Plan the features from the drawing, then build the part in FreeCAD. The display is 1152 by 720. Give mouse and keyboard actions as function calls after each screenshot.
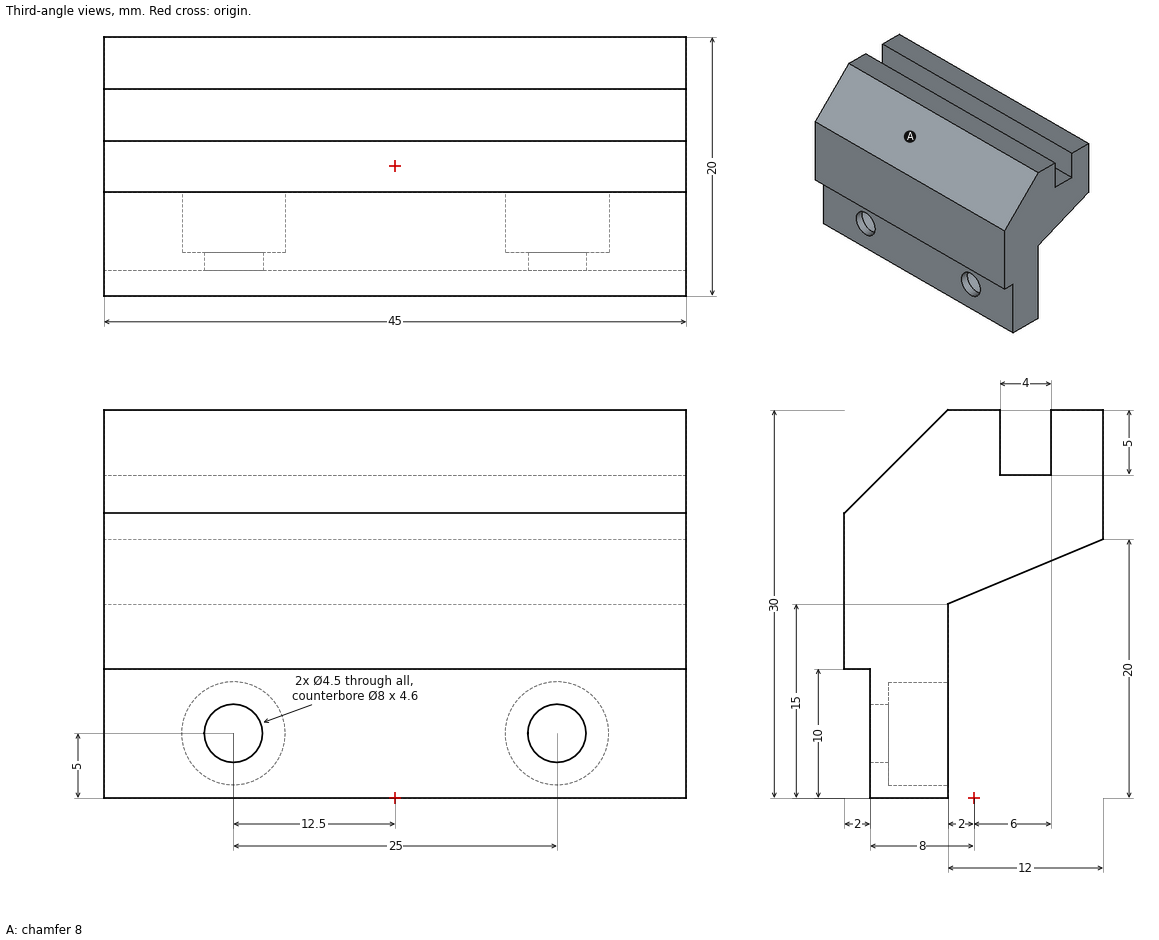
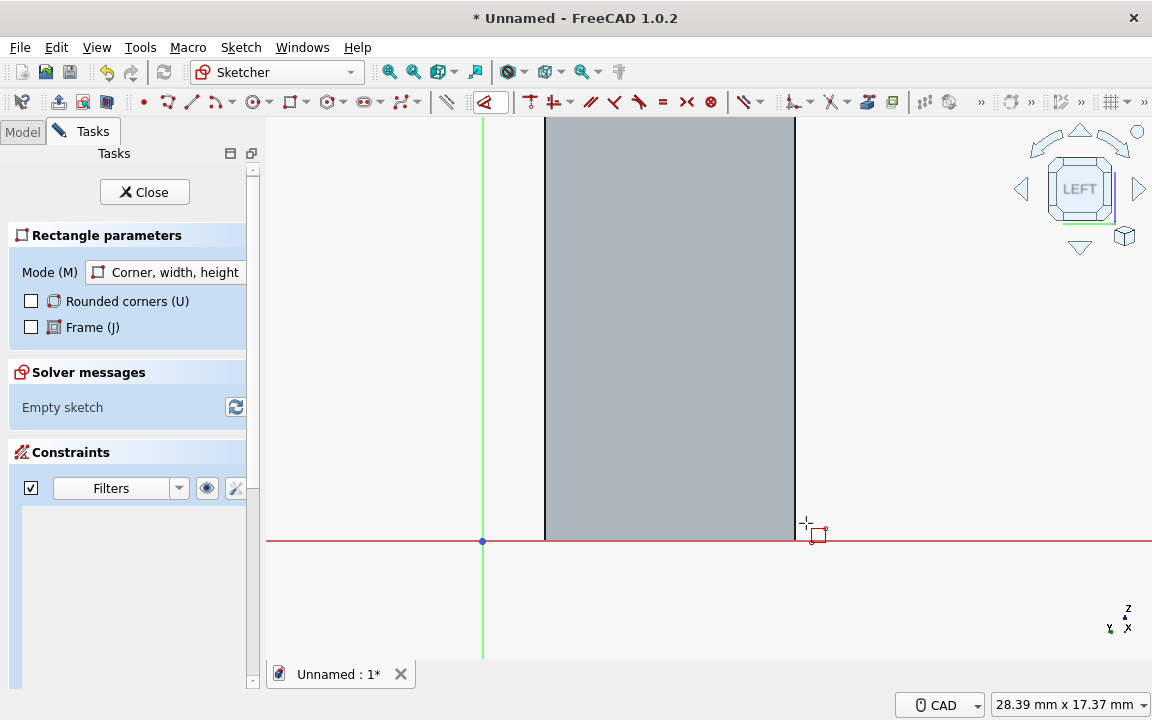
click(732, 229)
click(795, 541)
key(Escape)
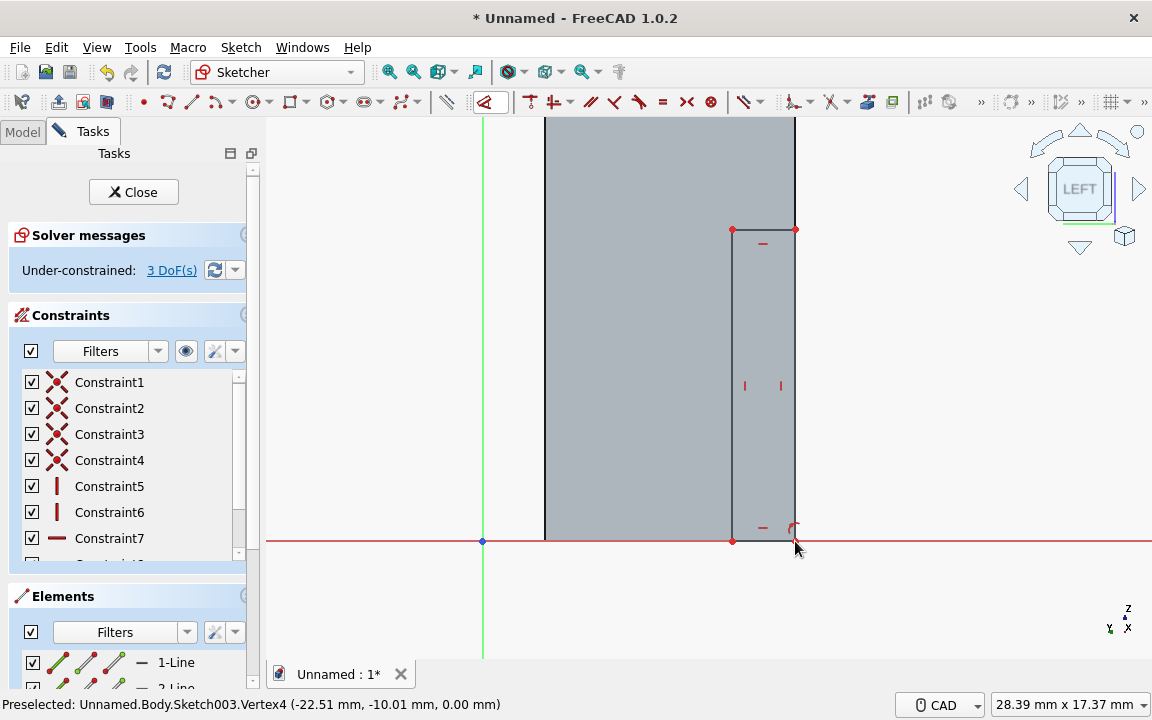
click(751, 541)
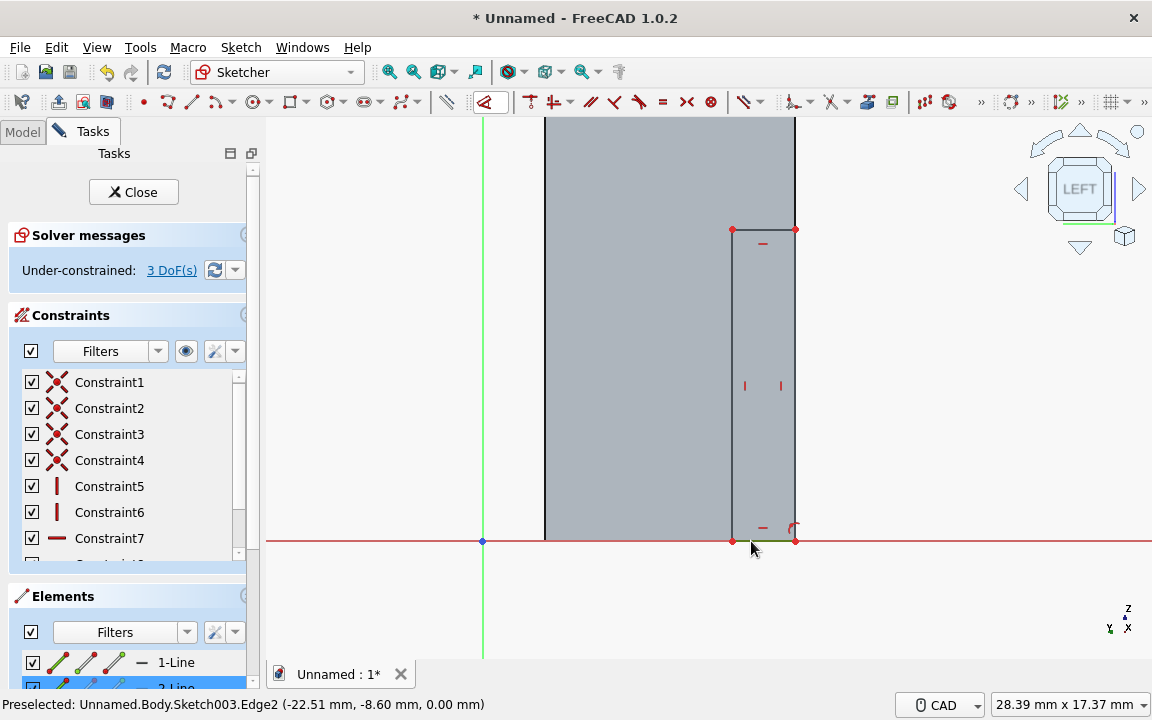
click(502, 102)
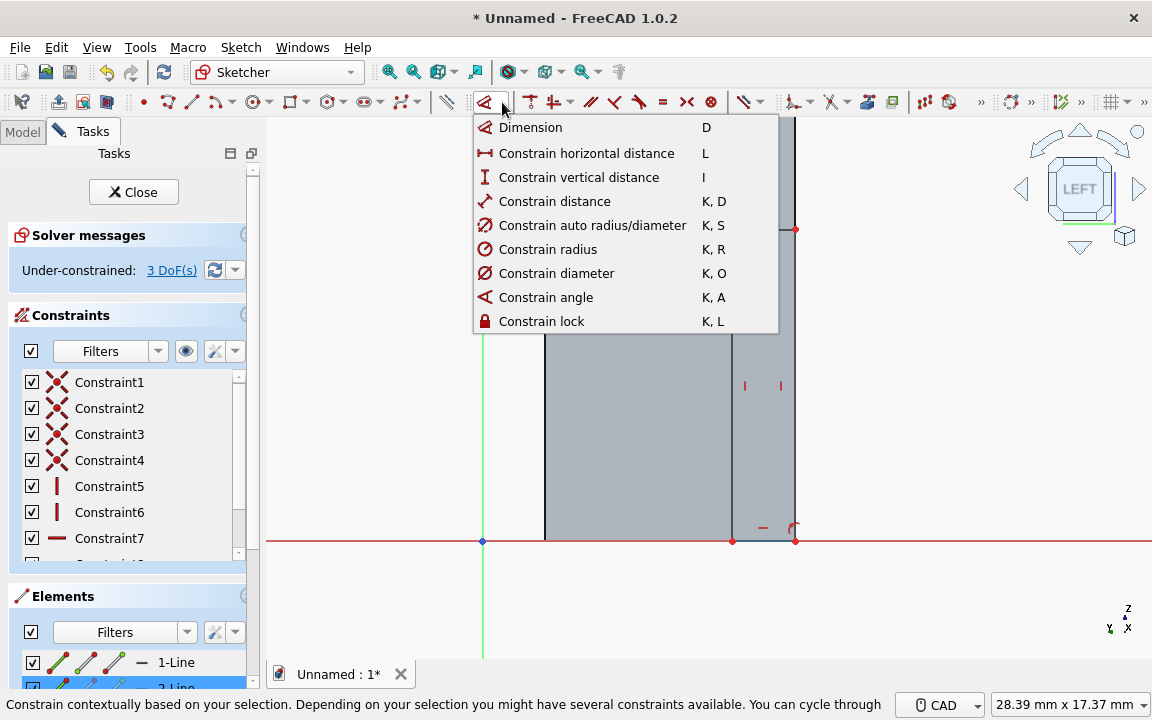
click(626, 153)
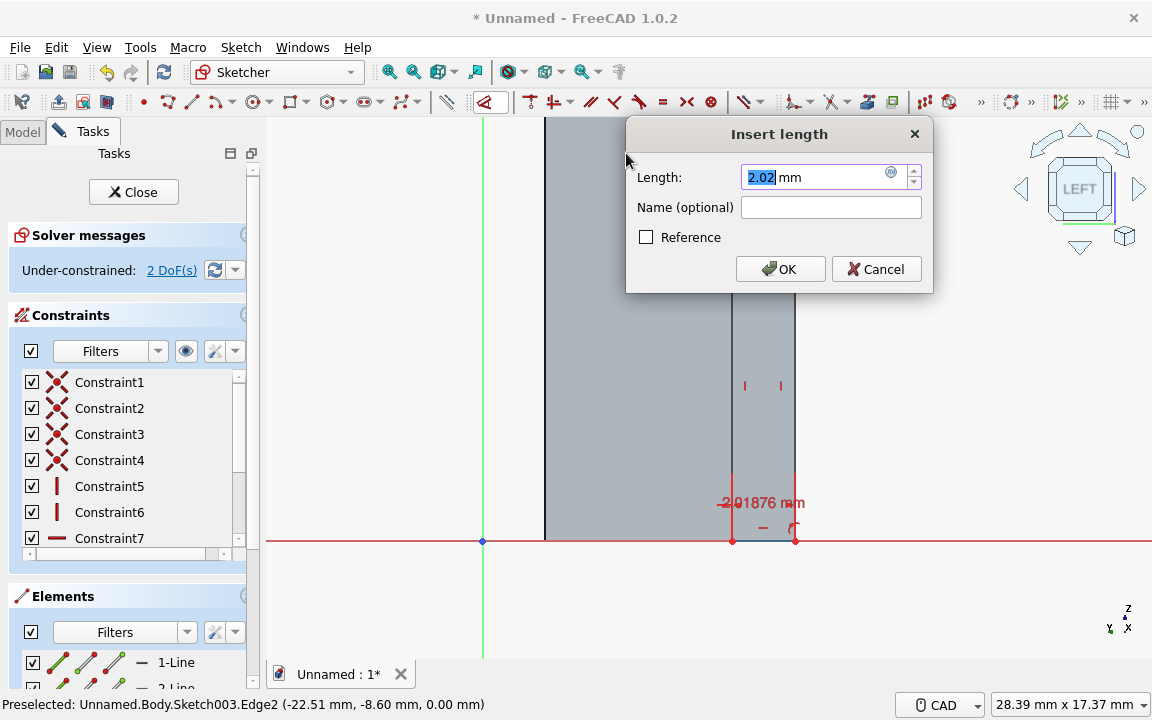
text(2)
key(Return)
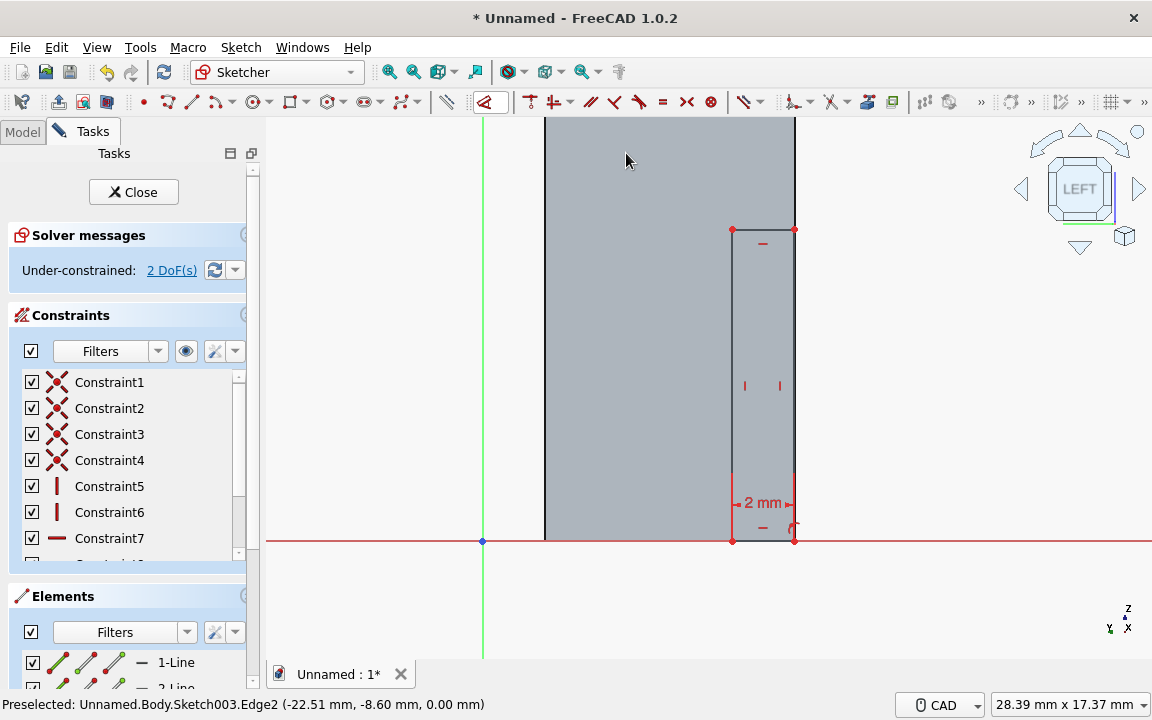
click(732, 323)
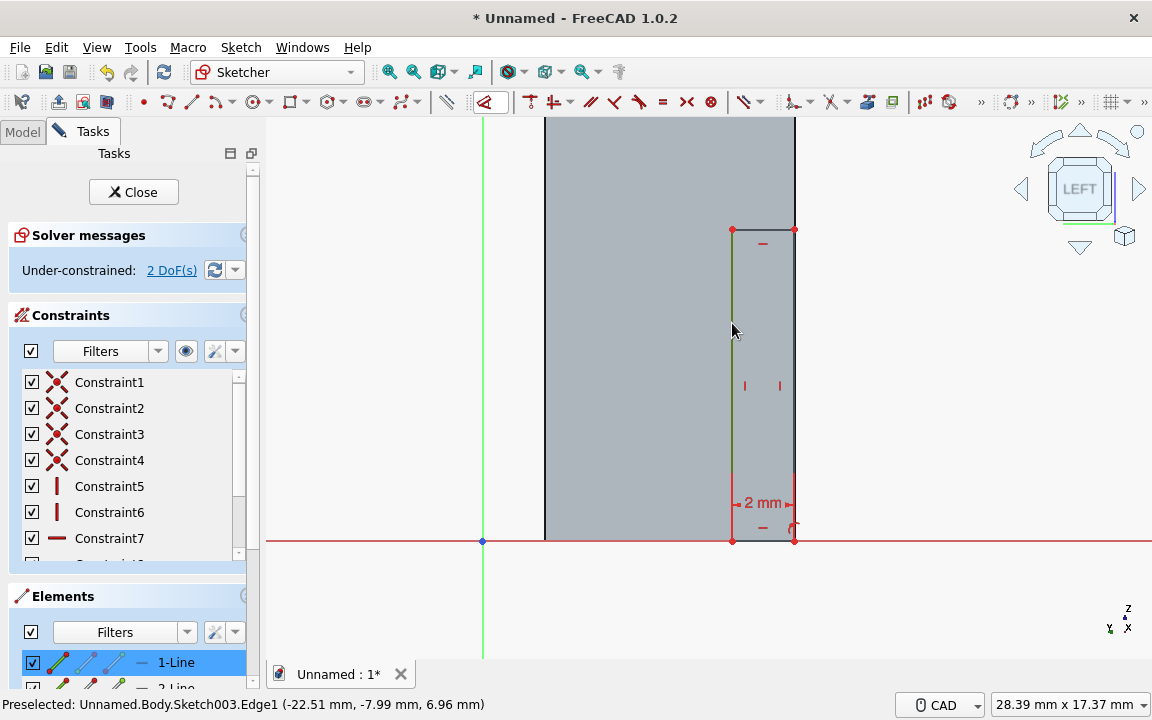
key(i)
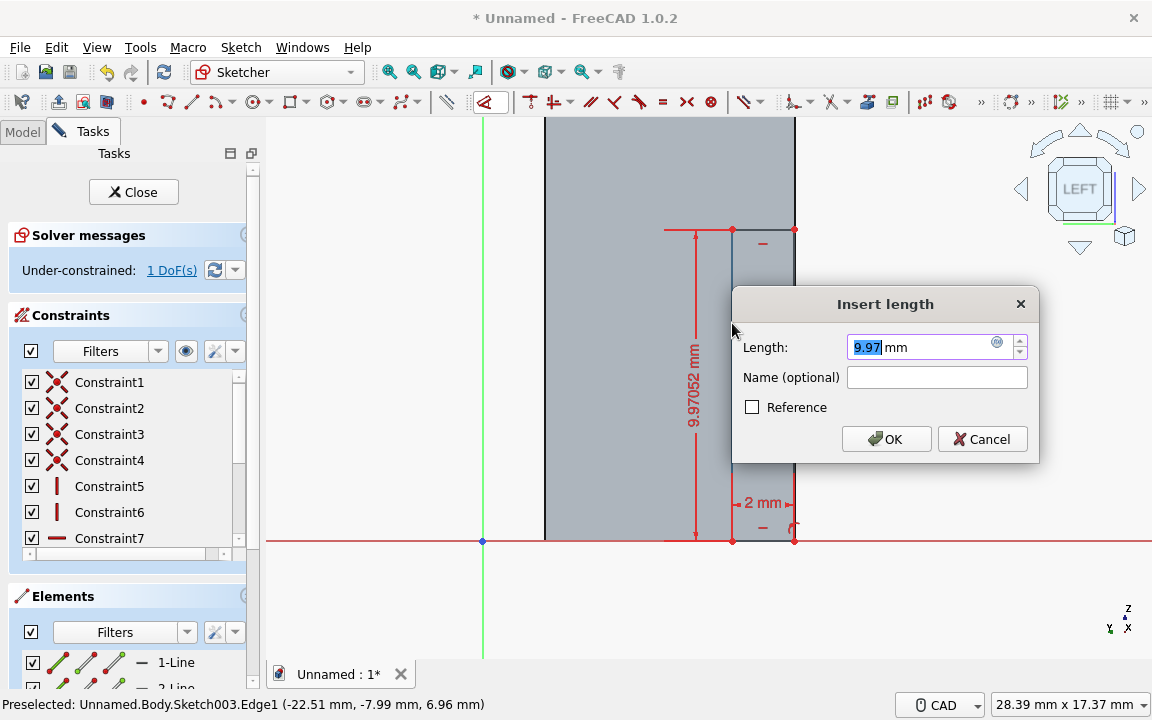
text(10)
key(Return)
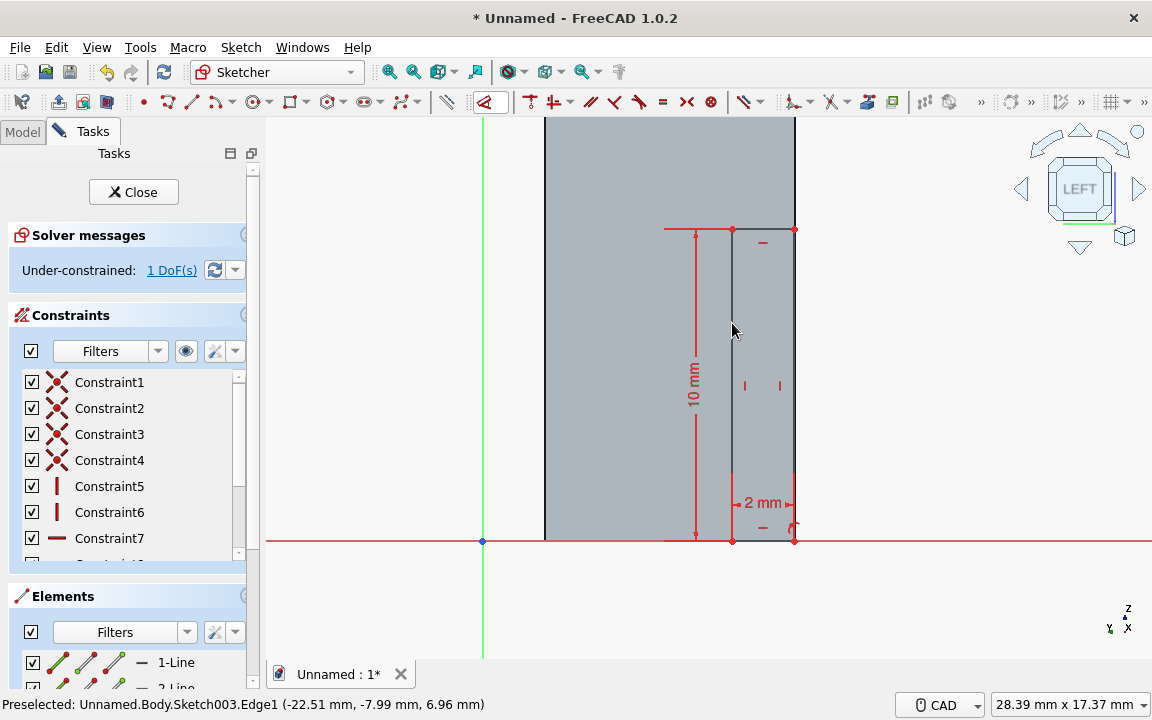
click(732, 229)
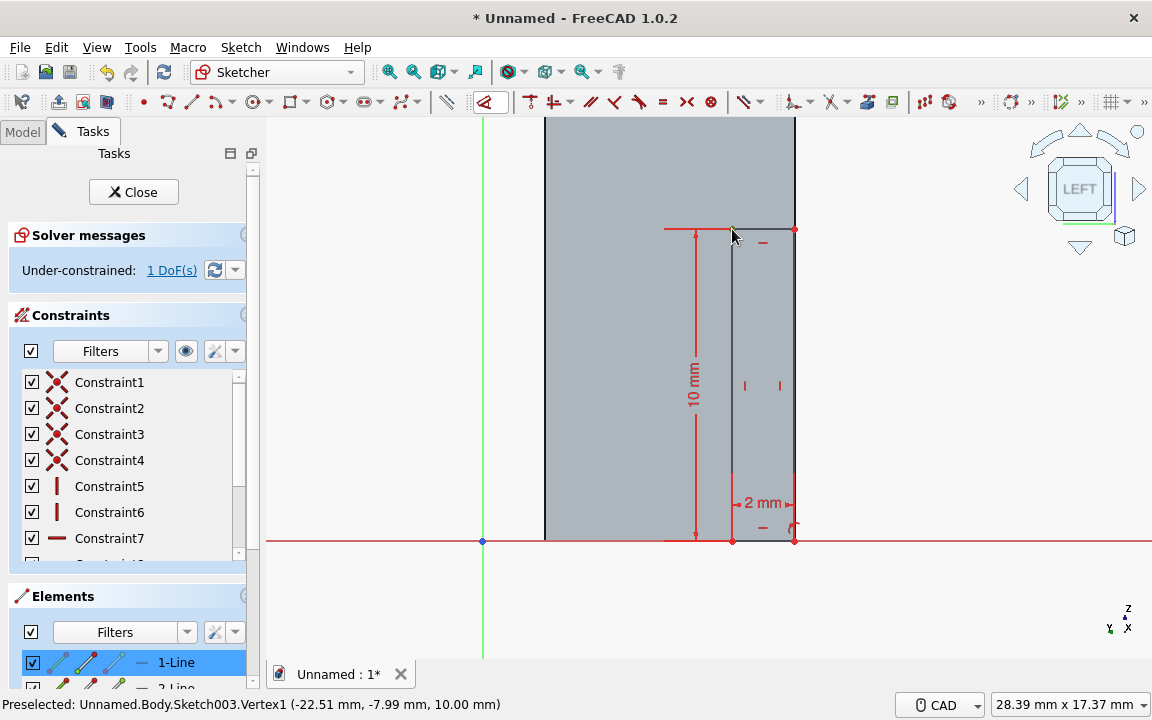
key(l)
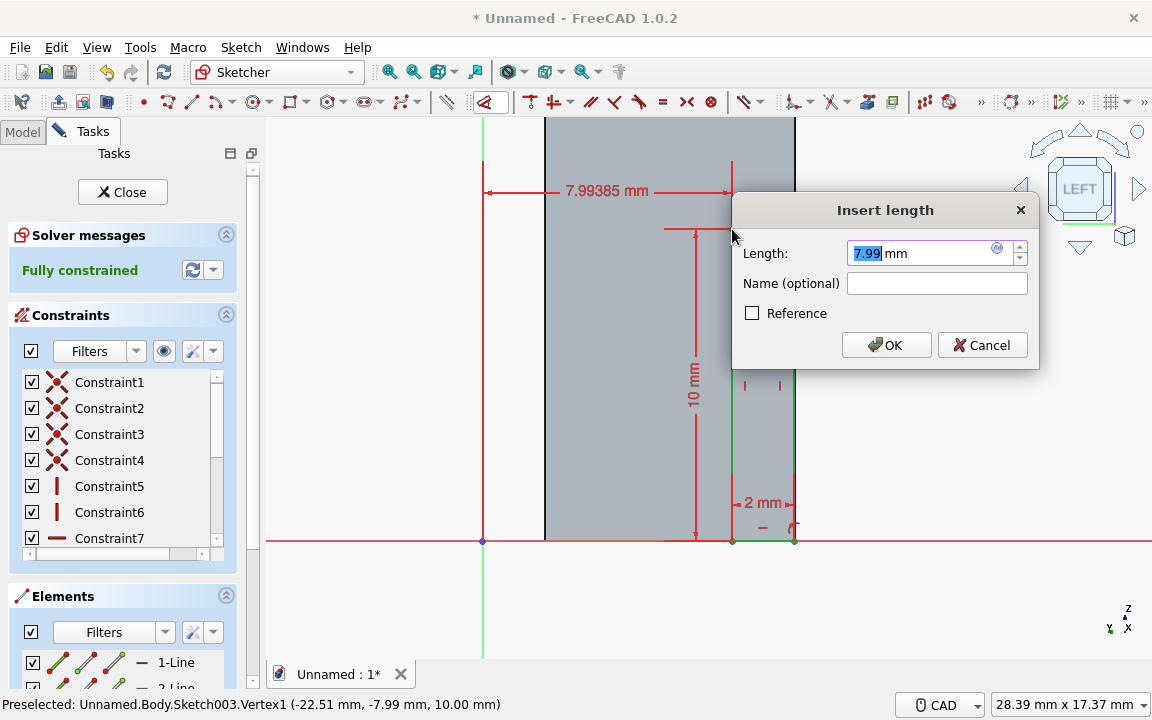
text(8)
key(Return)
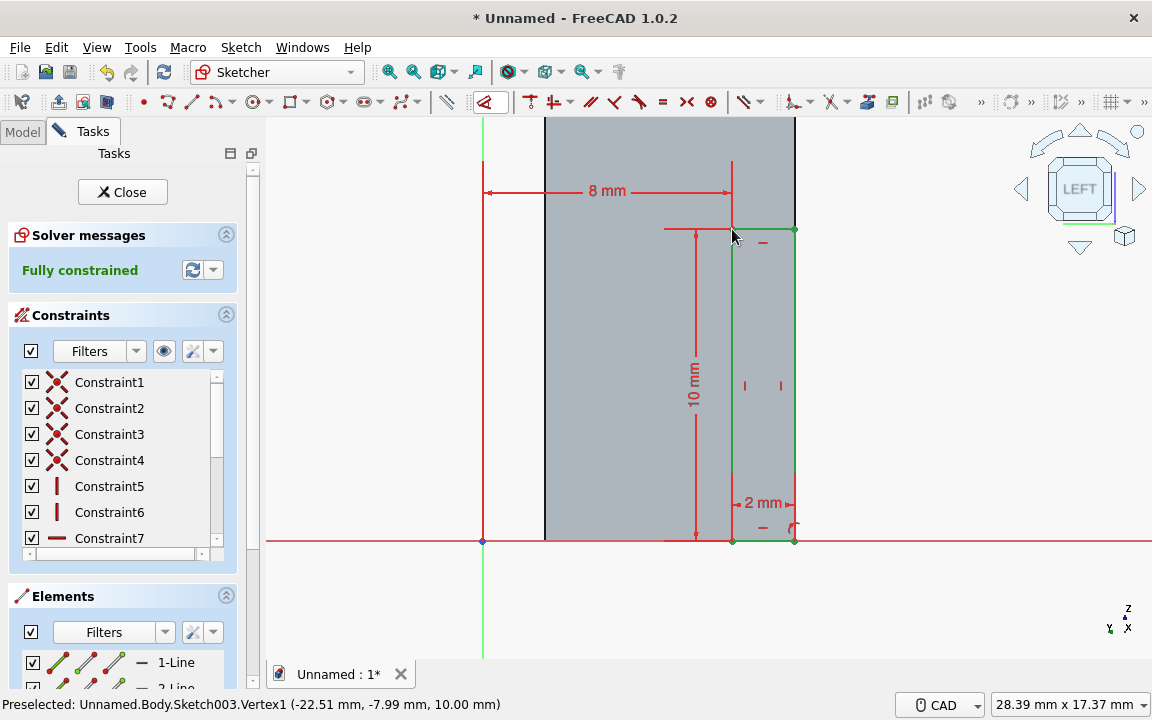
click(123, 192)